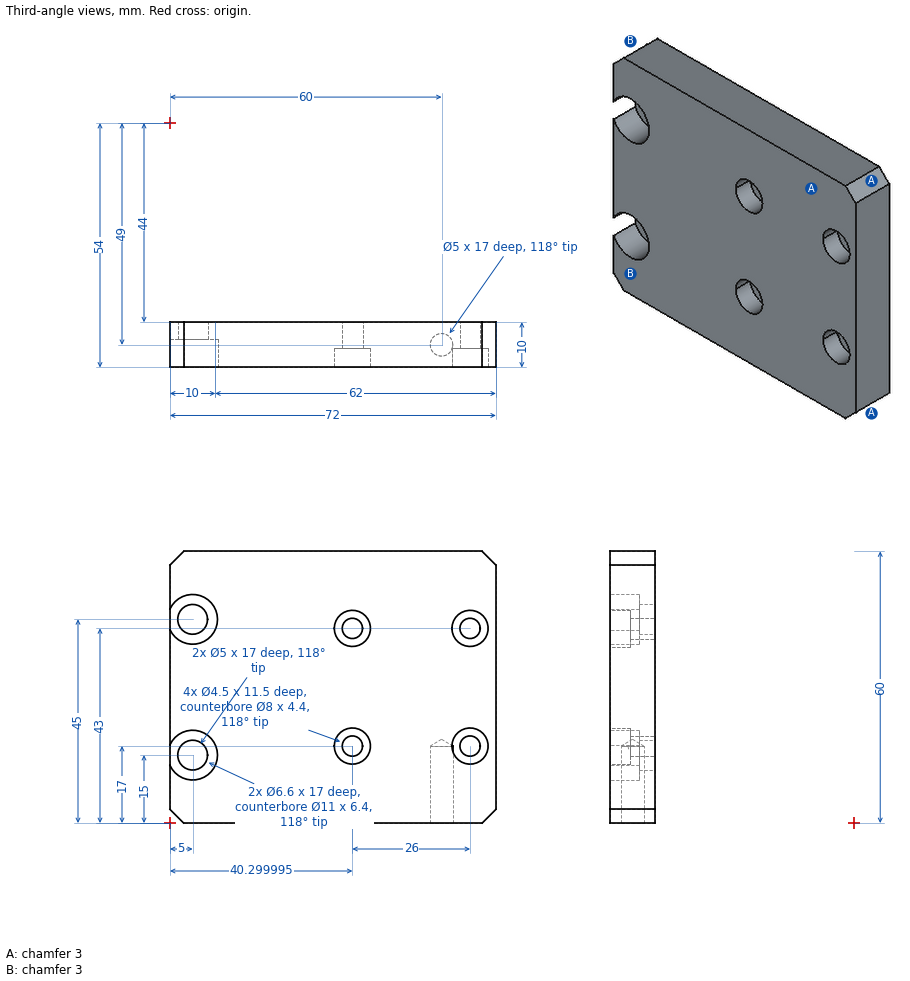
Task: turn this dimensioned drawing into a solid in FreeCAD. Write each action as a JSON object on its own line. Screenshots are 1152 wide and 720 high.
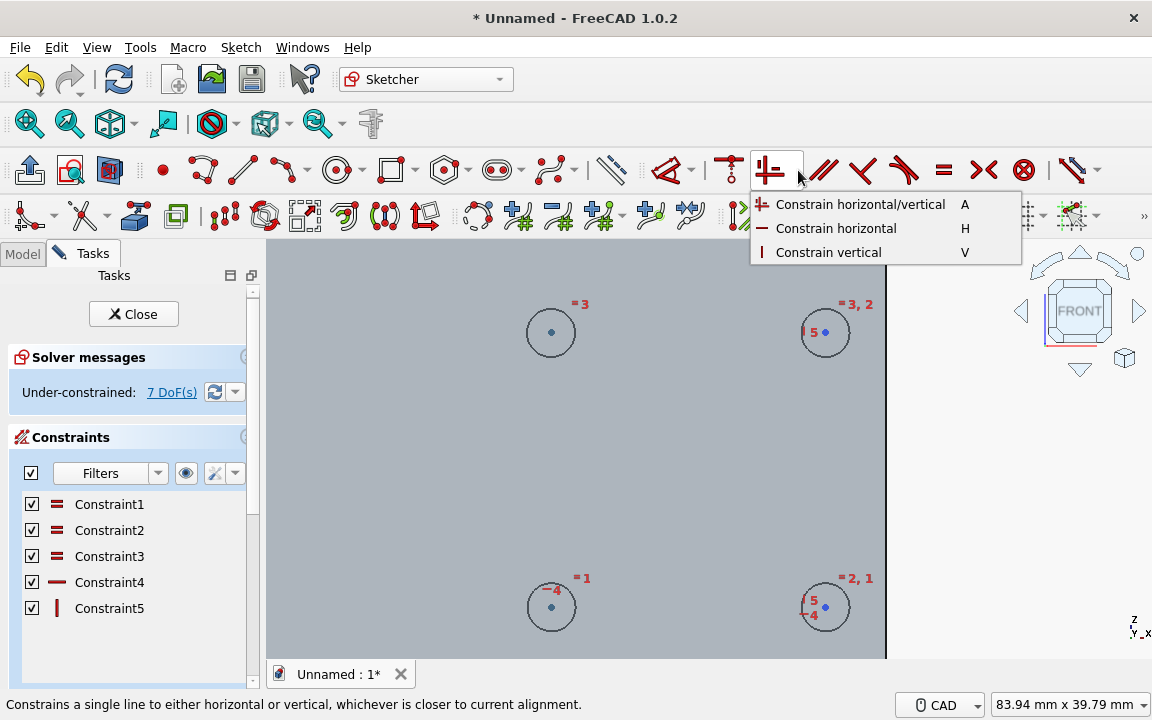
{"action": "left_click", "coordinate": [886, 252]}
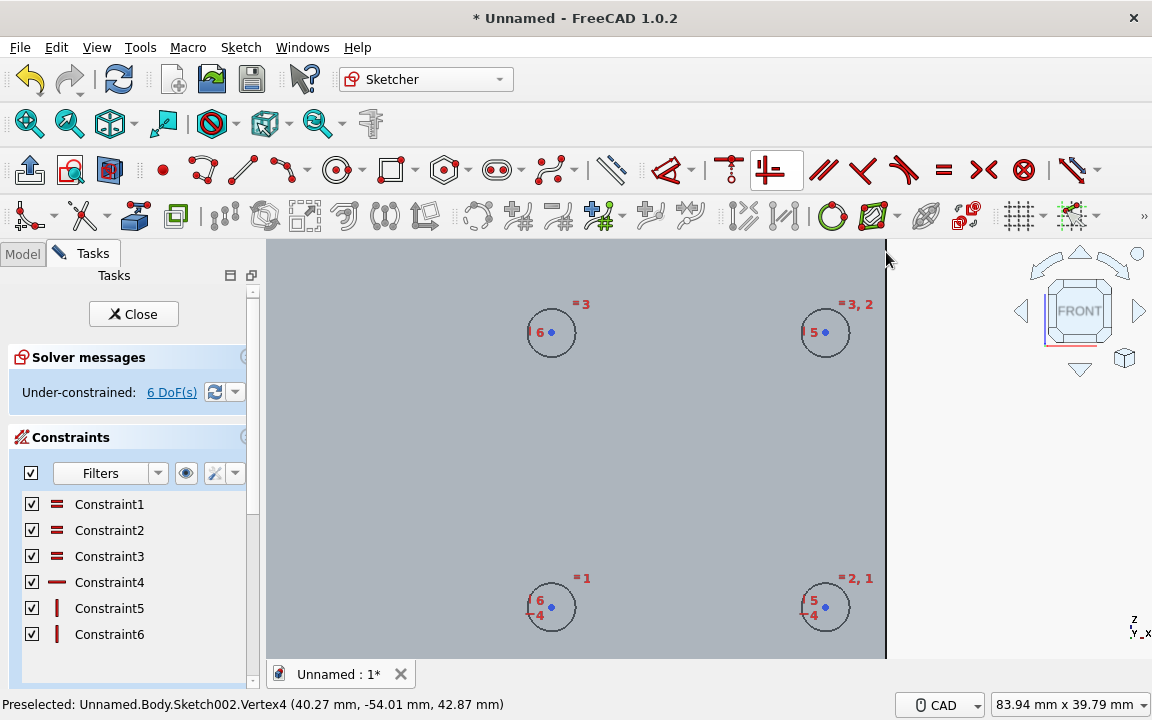
{"action": "left_click", "coordinate": [826, 333]}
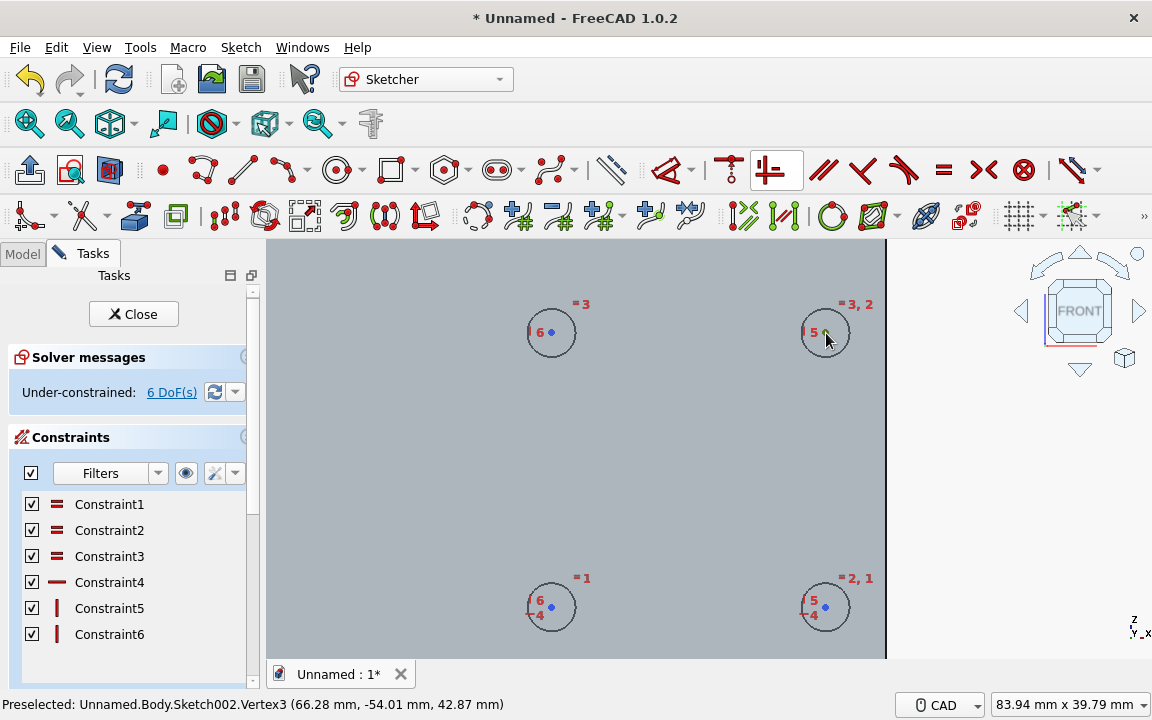
{"action": "left_click", "coordinate": [552, 333]}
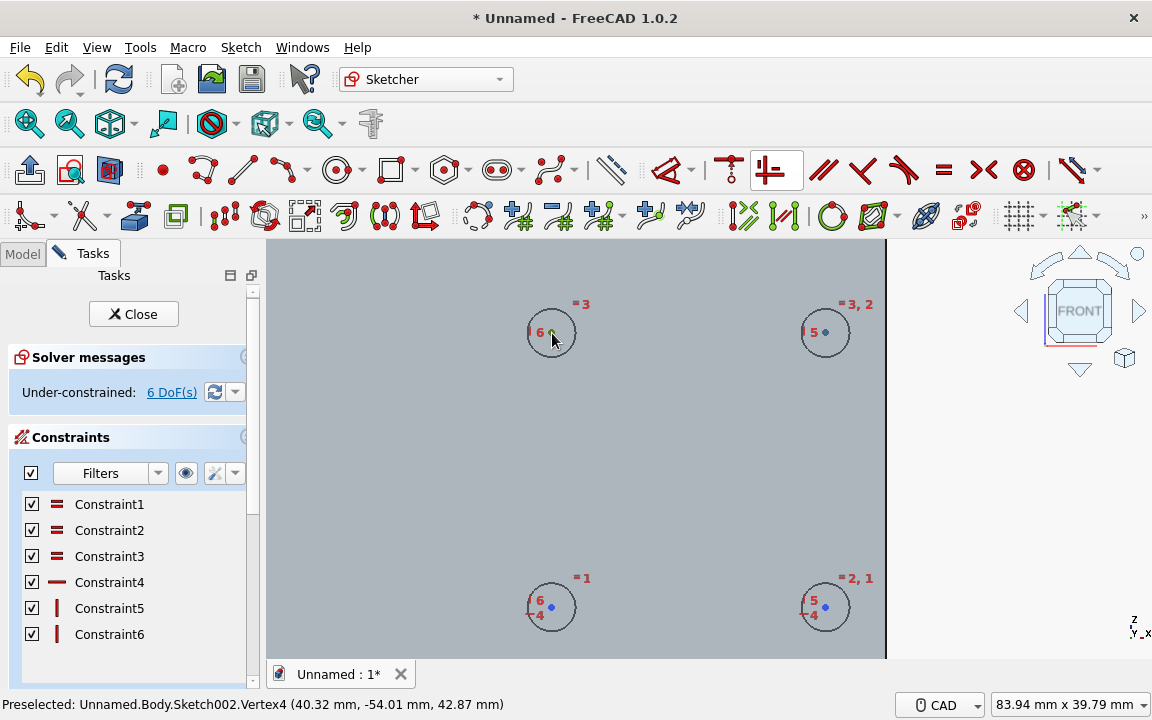
{"action": "left_click", "coordinate": [798, 170]}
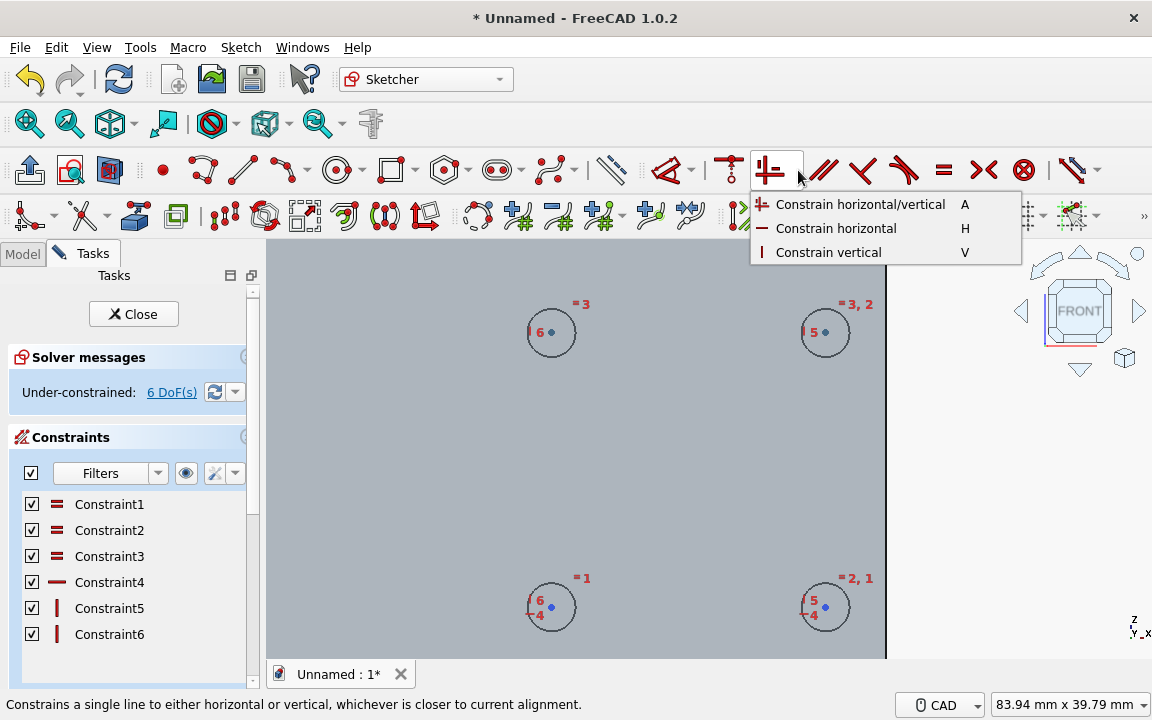
{"action": "left_click", "coordinate": [886, 228]}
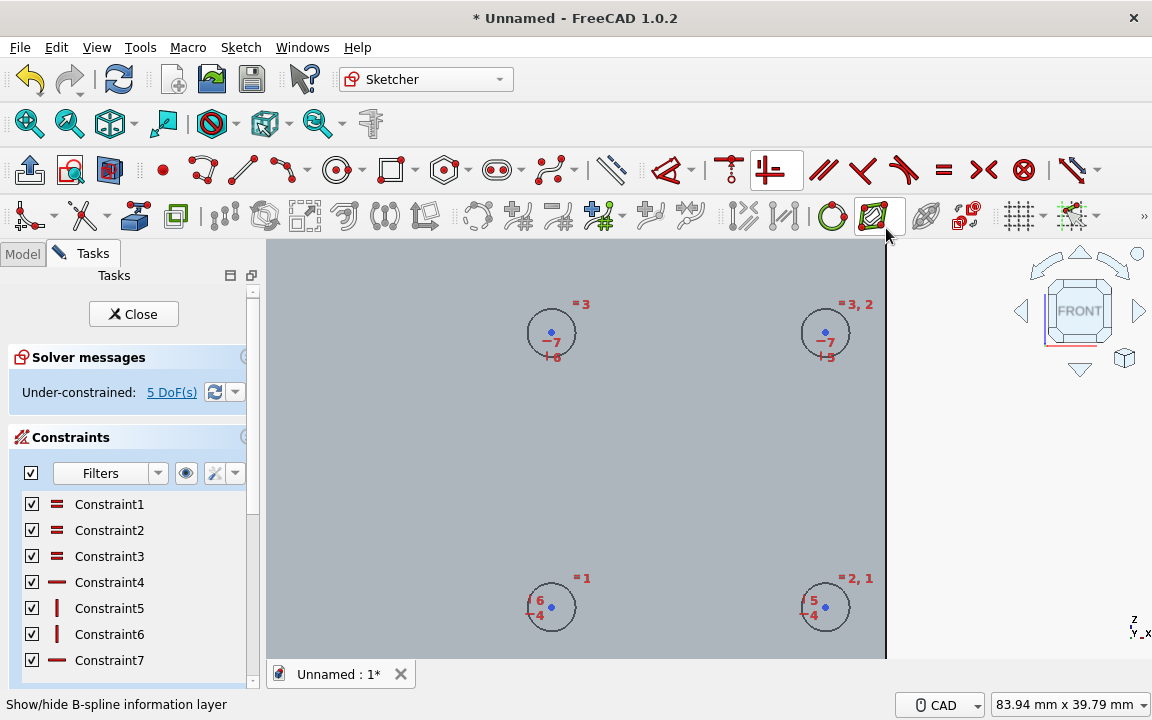
{"action": "left_click", "coordinate": [666, 170]}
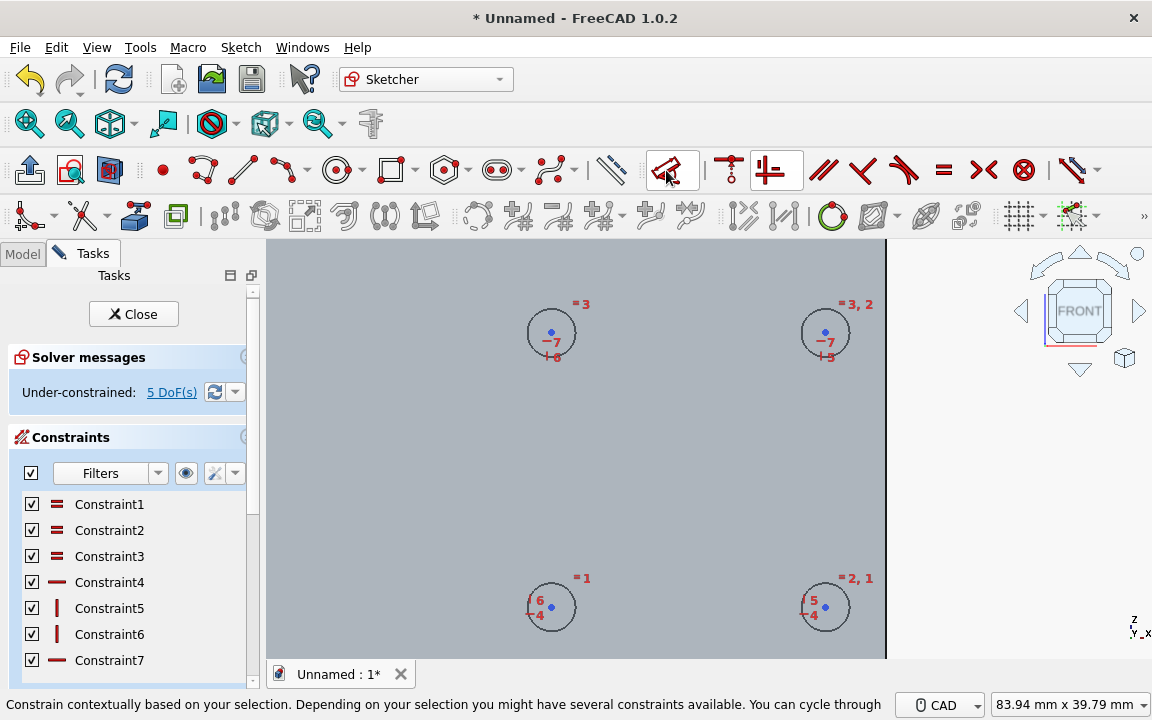
{"action": "left_click", "coordinate": [568, 590]}
{"action": "left_click", "coordinate": [590, 567]}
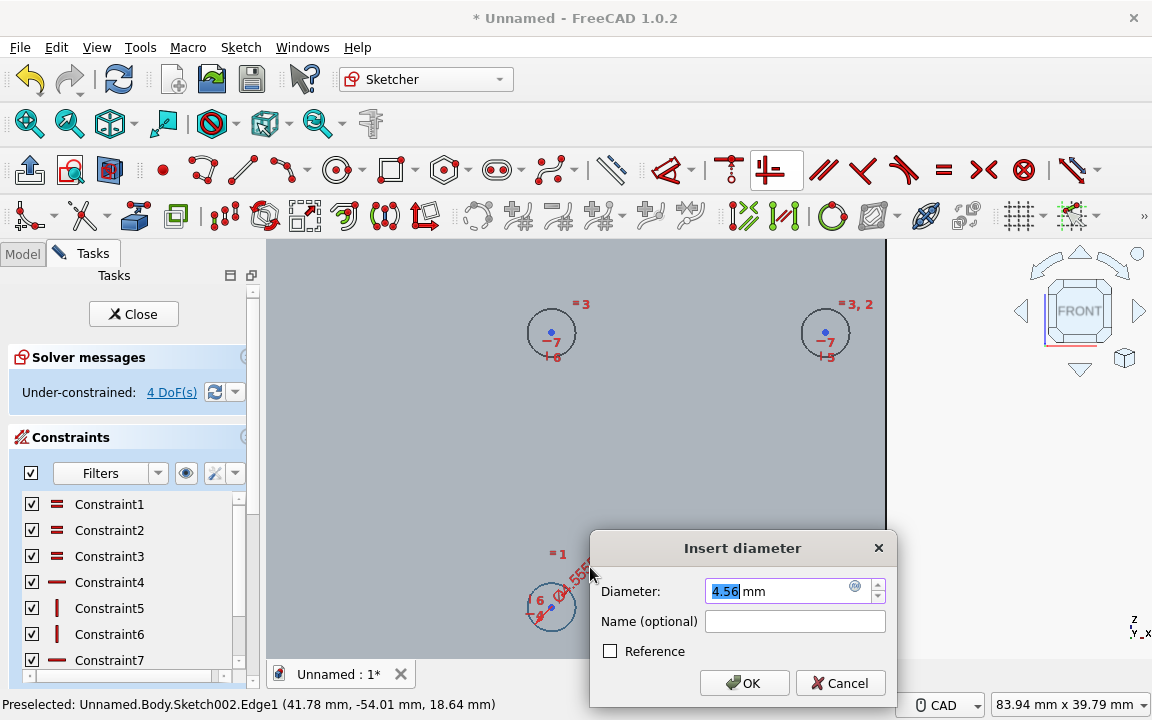
{"action": "type", "text": "4.5"}
{"action": "key", "text": "Return"}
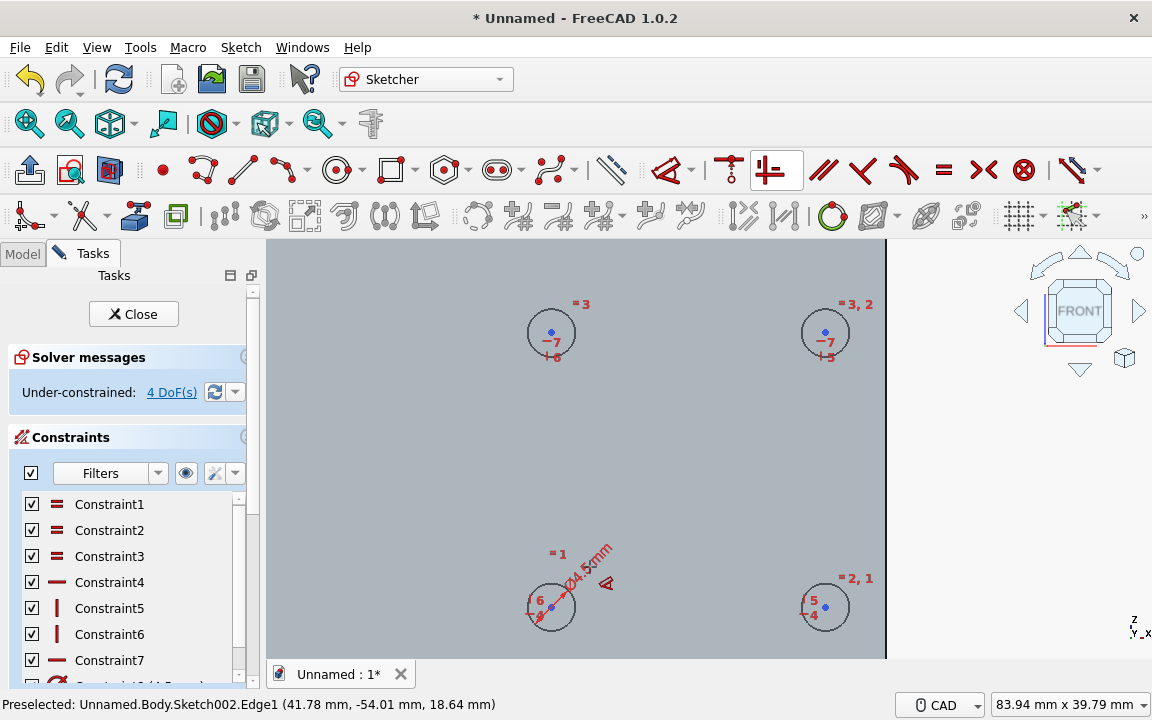
{"action": "left_click", "coordinate": [552, 607]}
{"action": "left_click", "coordinate": [586, 625]}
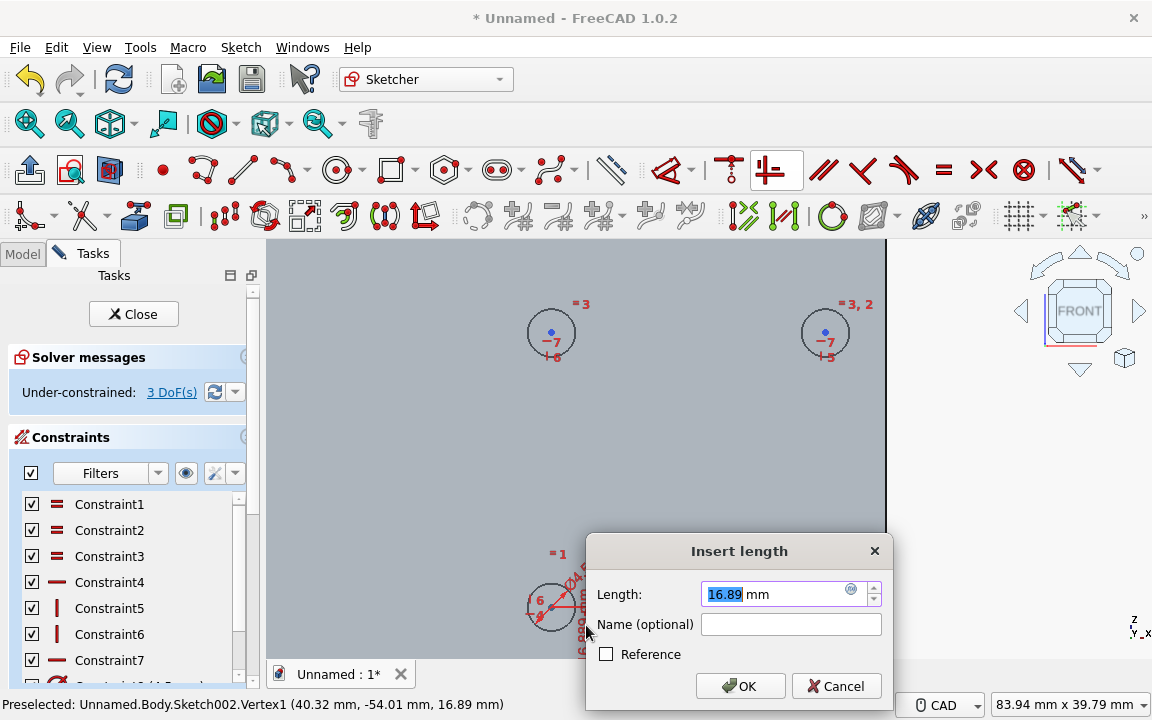
{"action": "type", "text": "17"}
{"action": "key", "text": "Return"}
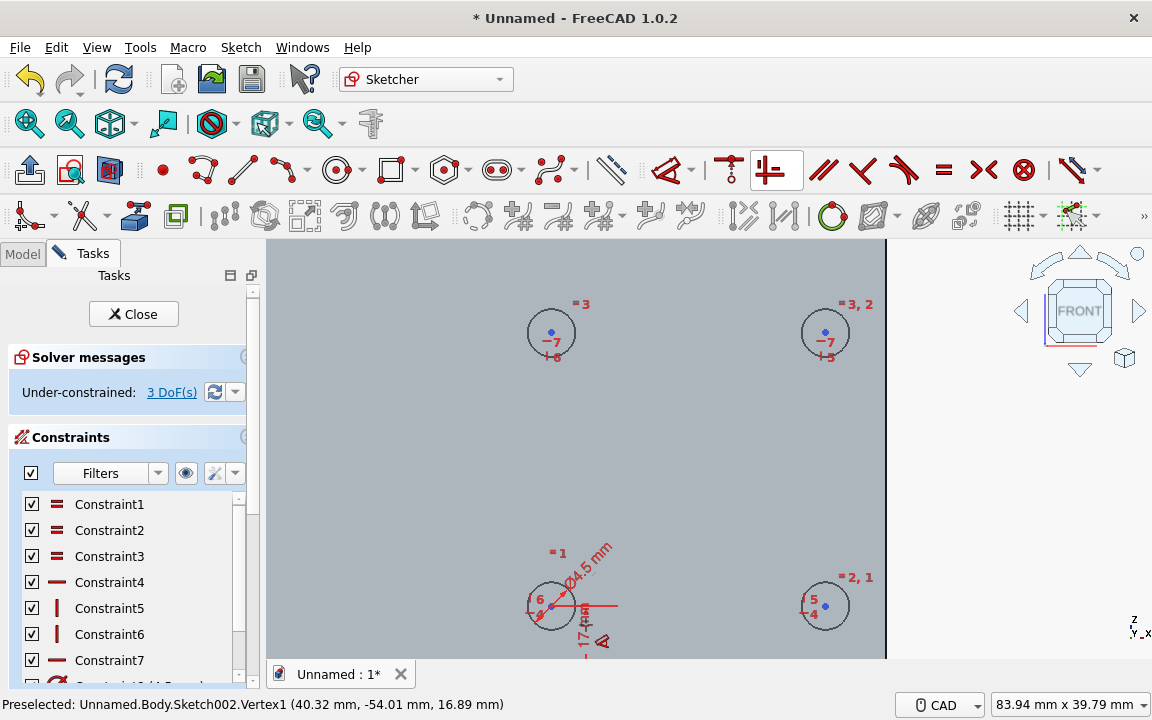
{"action": "left_click", "coordinate": [826, 333]}
{"action": "left_click", "coordinate": [860, 482]}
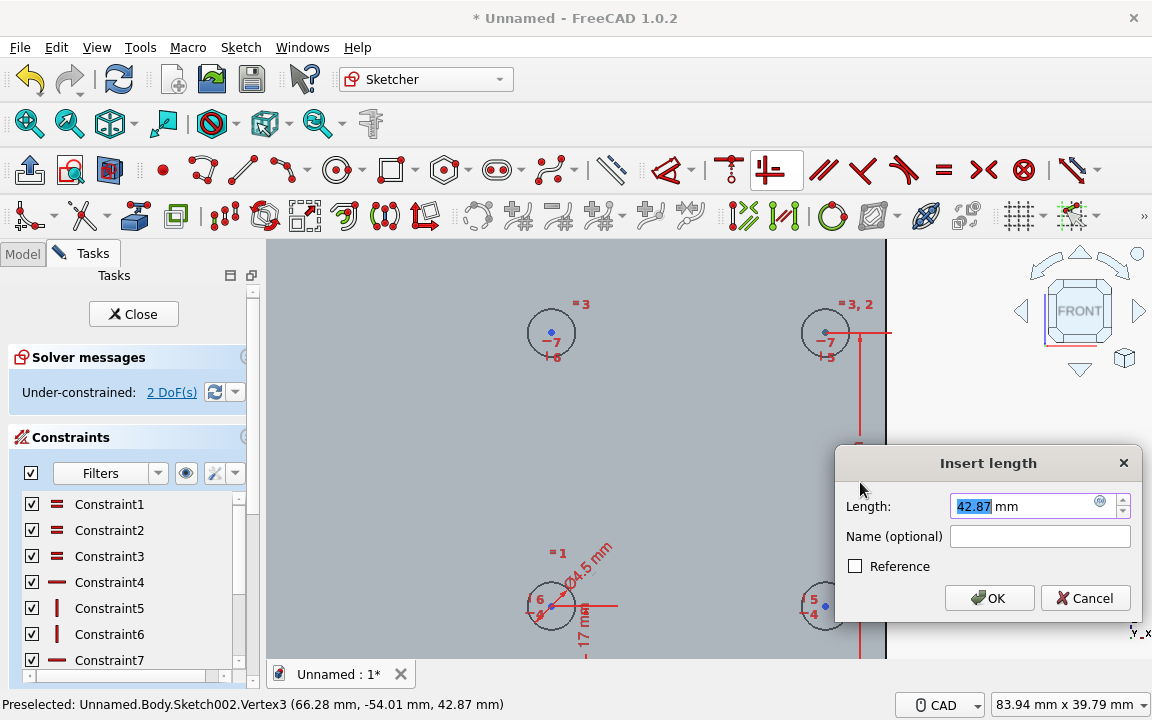
{"action": "type", "text": "43"}
{"action": "key", "text": "Return"}